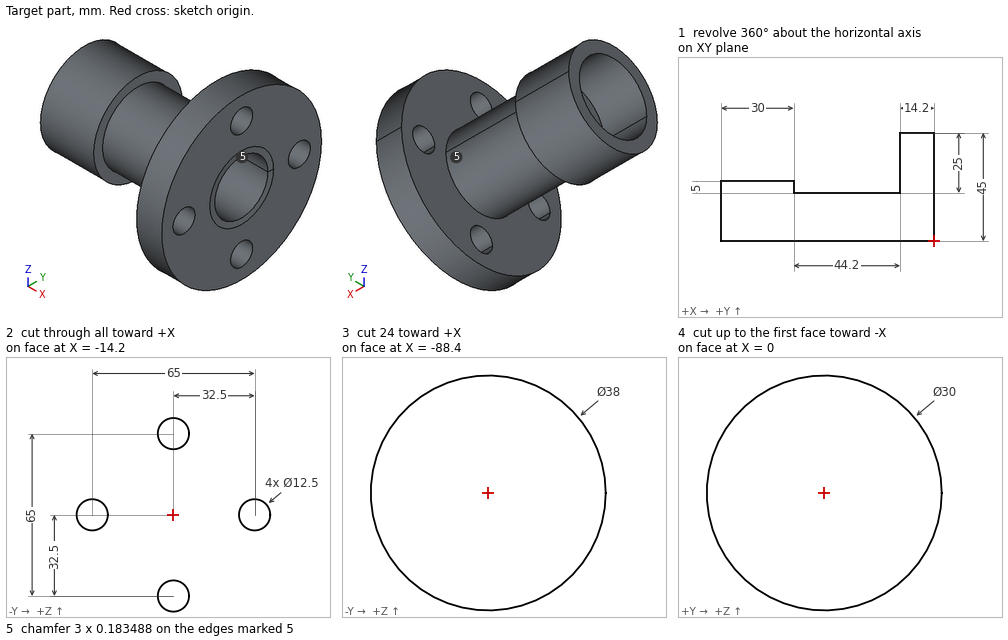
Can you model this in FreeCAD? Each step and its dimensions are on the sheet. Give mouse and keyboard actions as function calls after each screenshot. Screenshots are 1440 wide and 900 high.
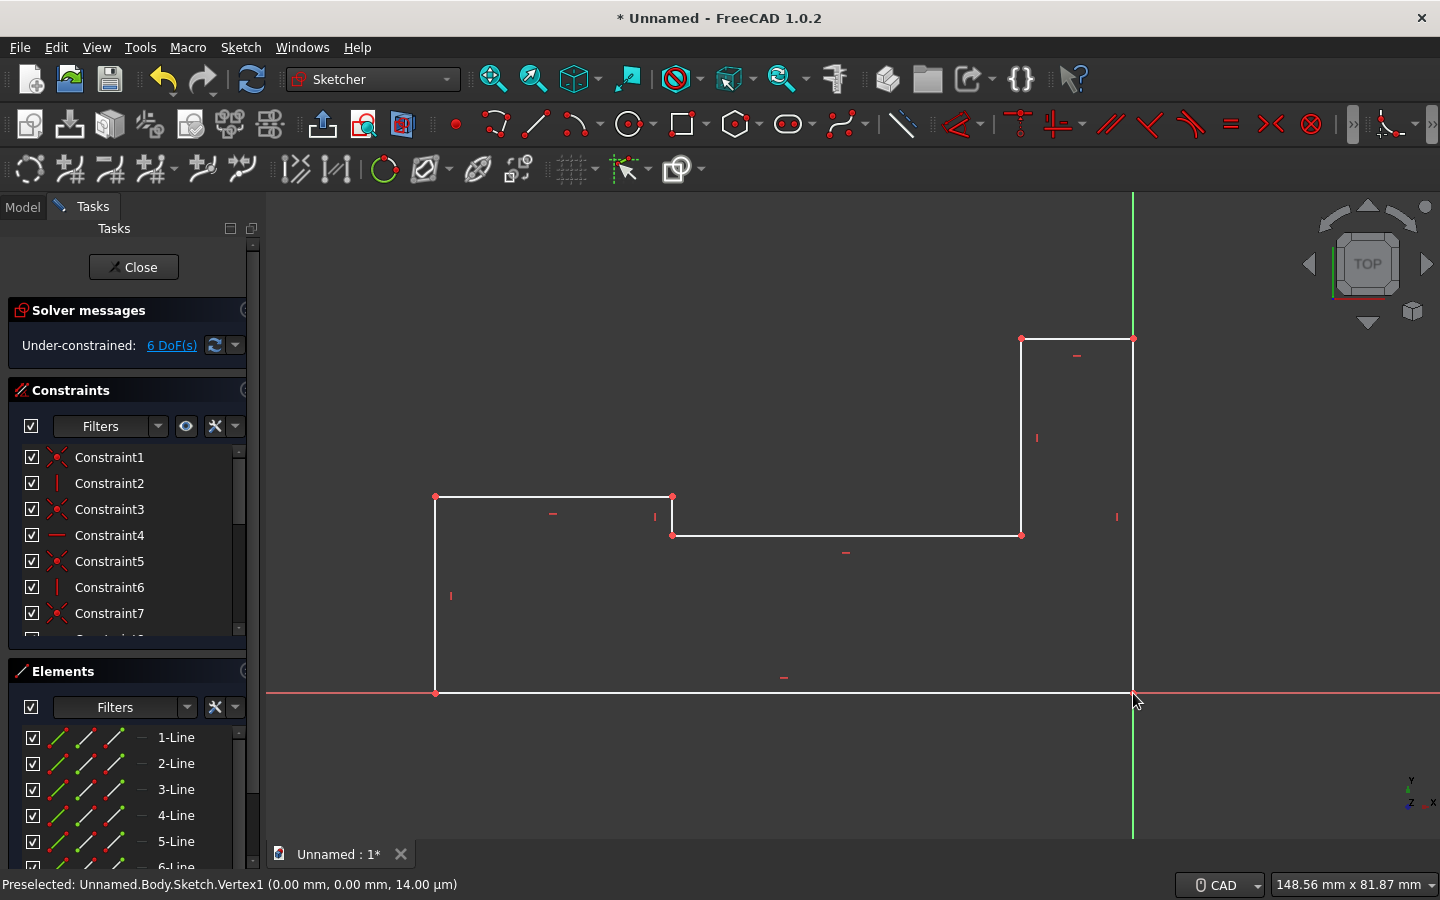
click(956, 124)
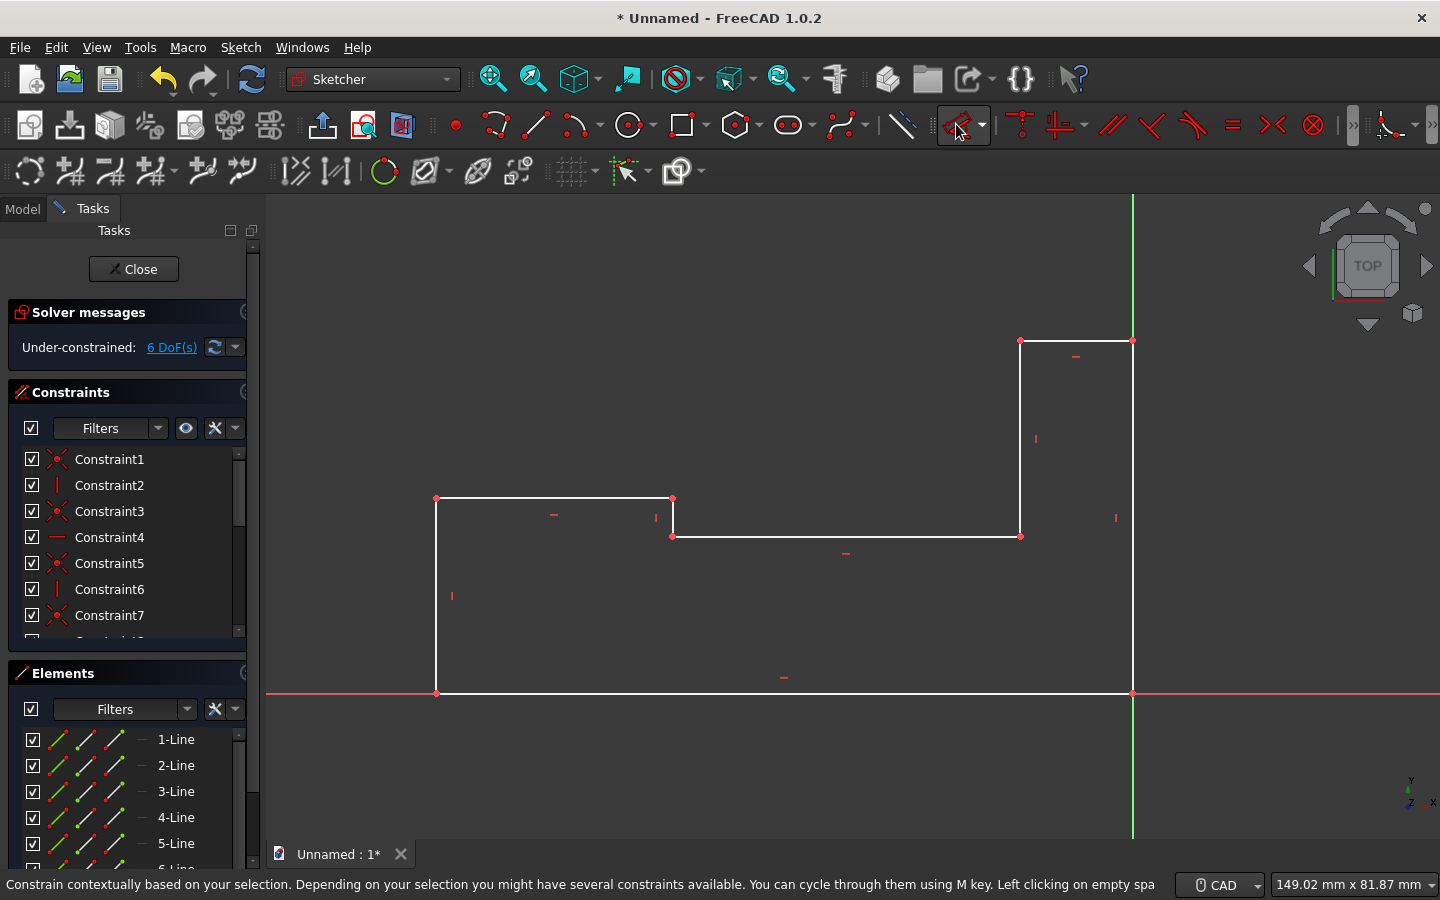
click(673, 525)
click(639, 517)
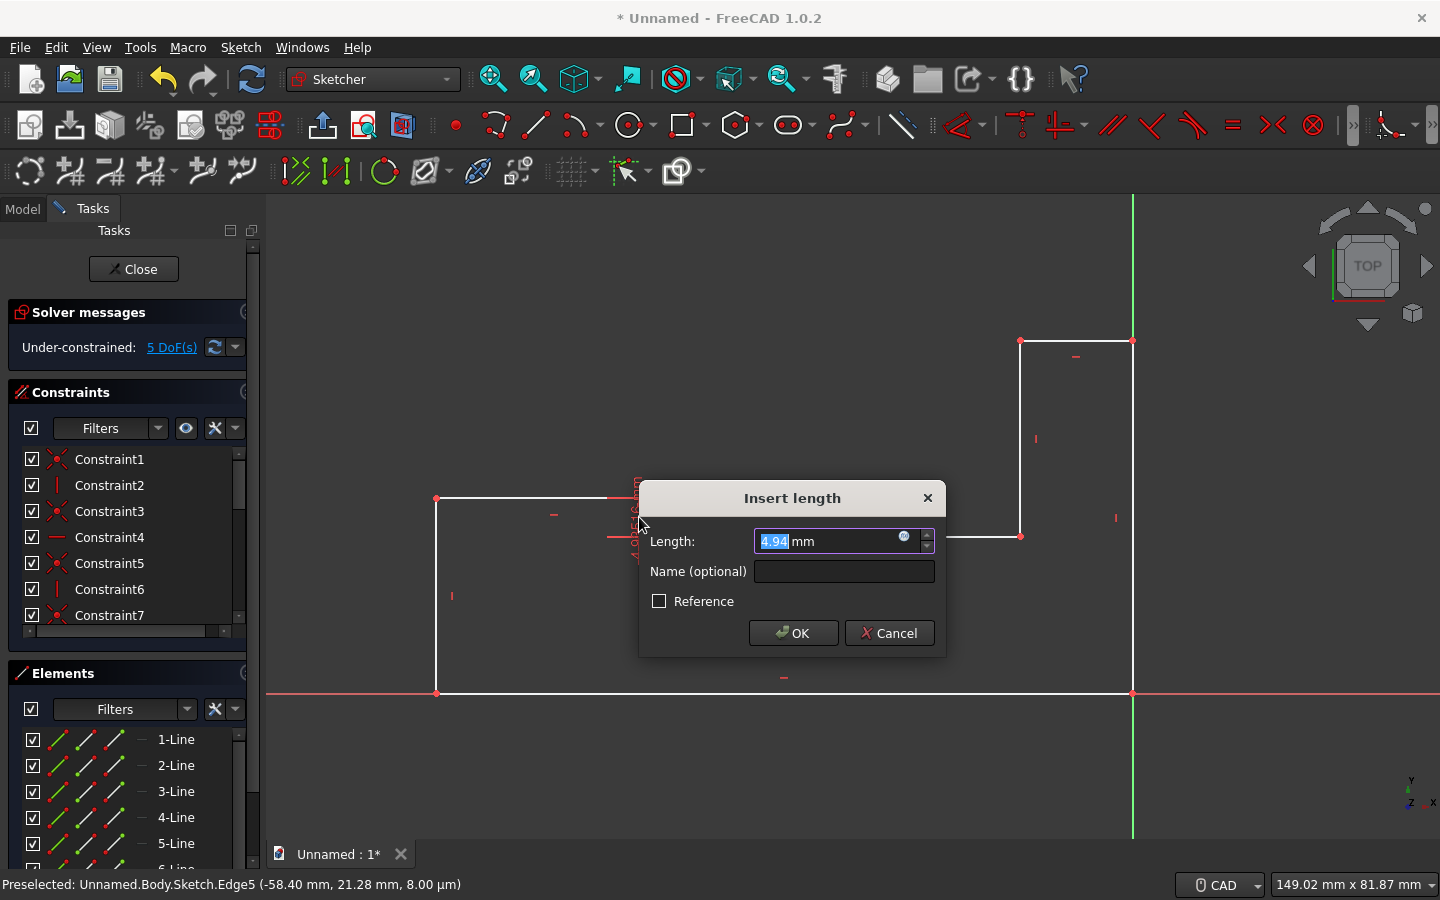
text(5)
key(Return)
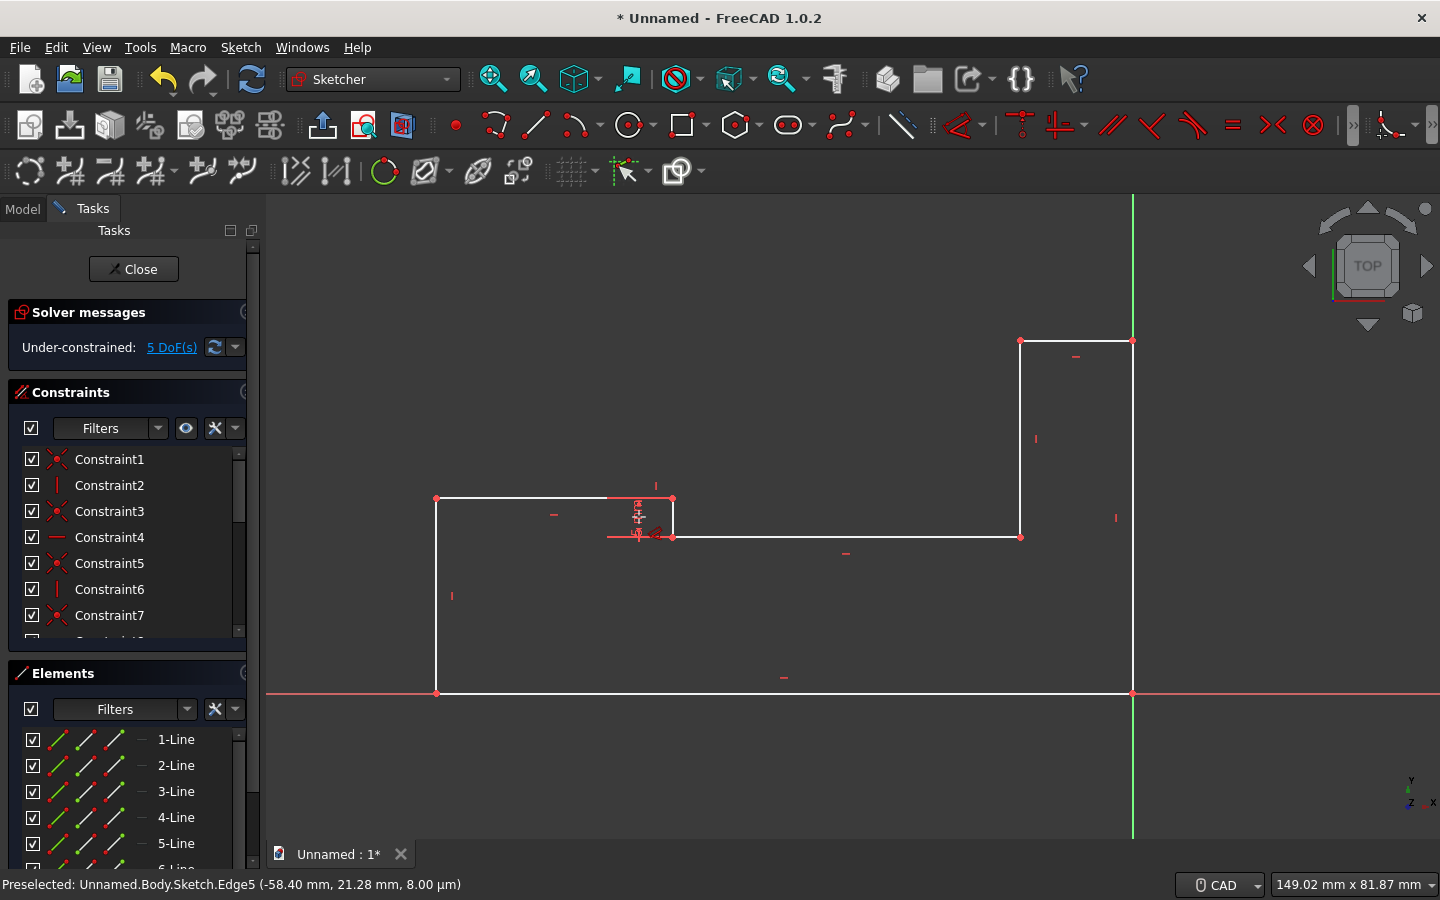
click(1133, 588)
click(1167, 517)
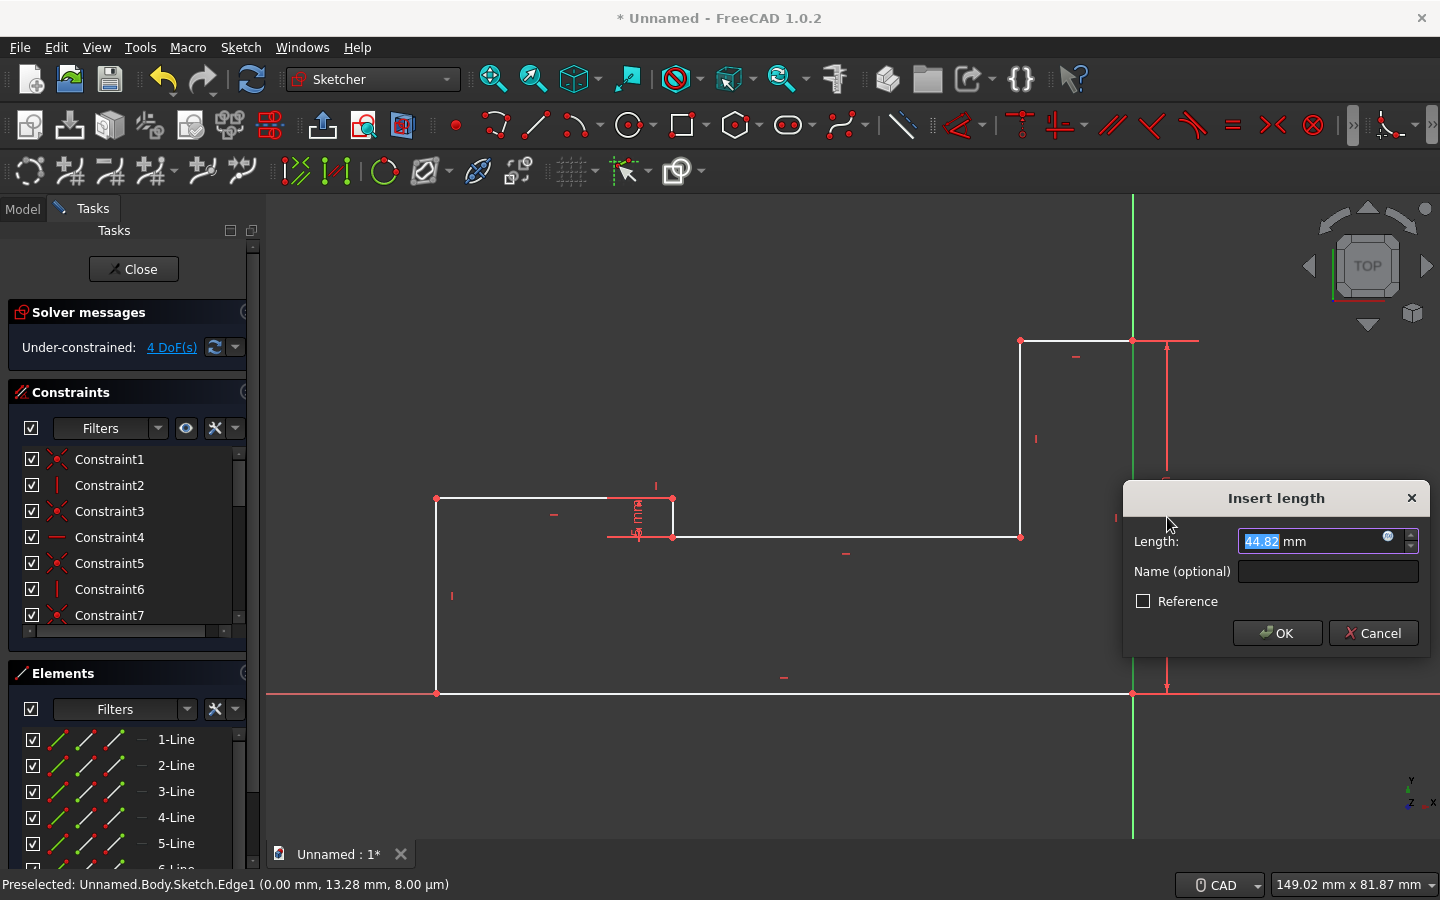
text(45)
key(Return)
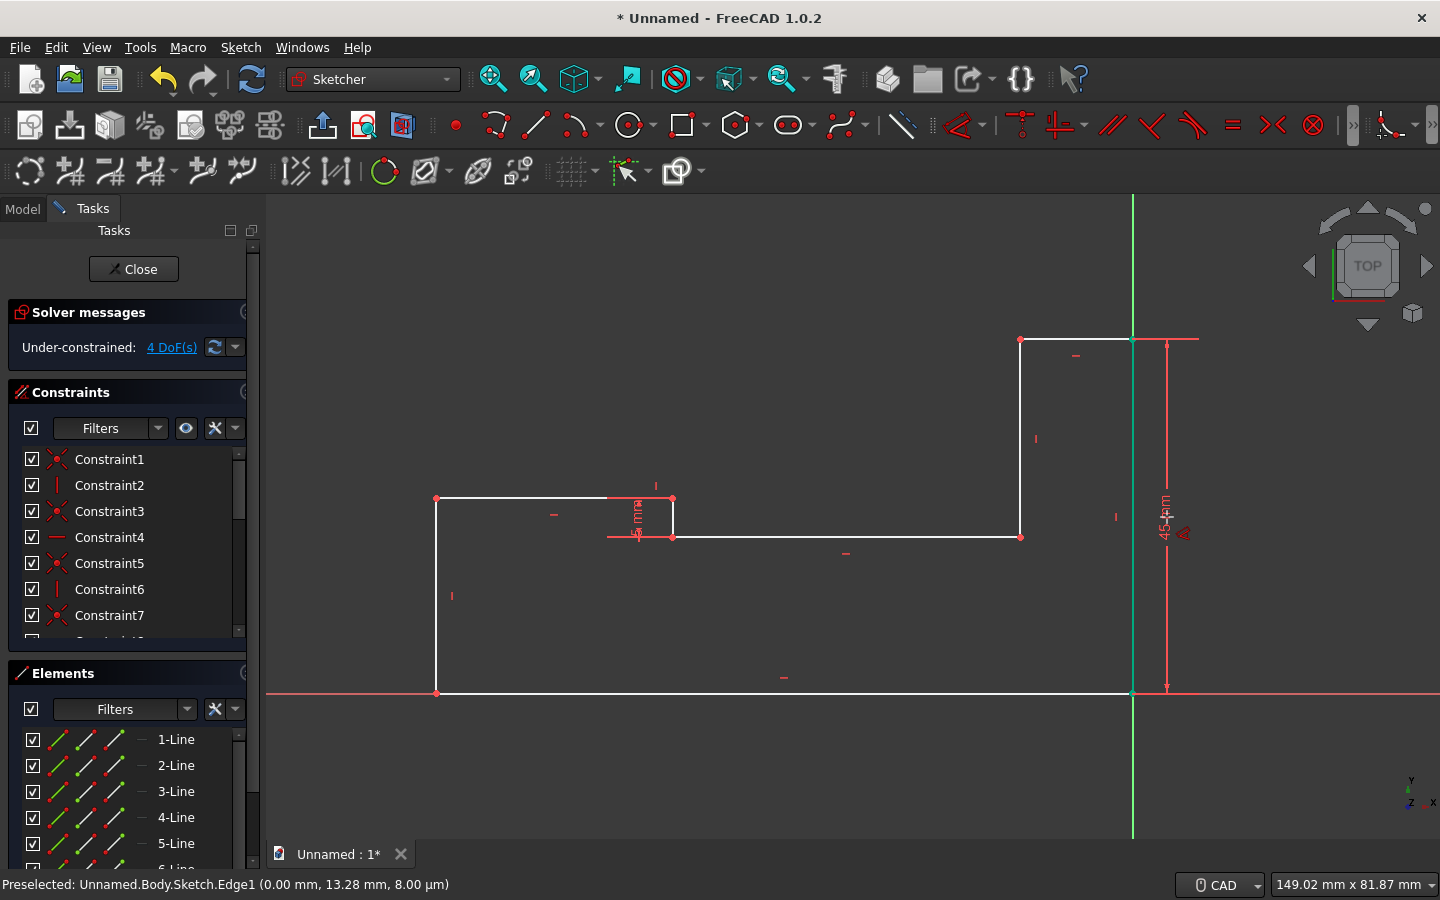
click(1020, 399)
click(1054, 438)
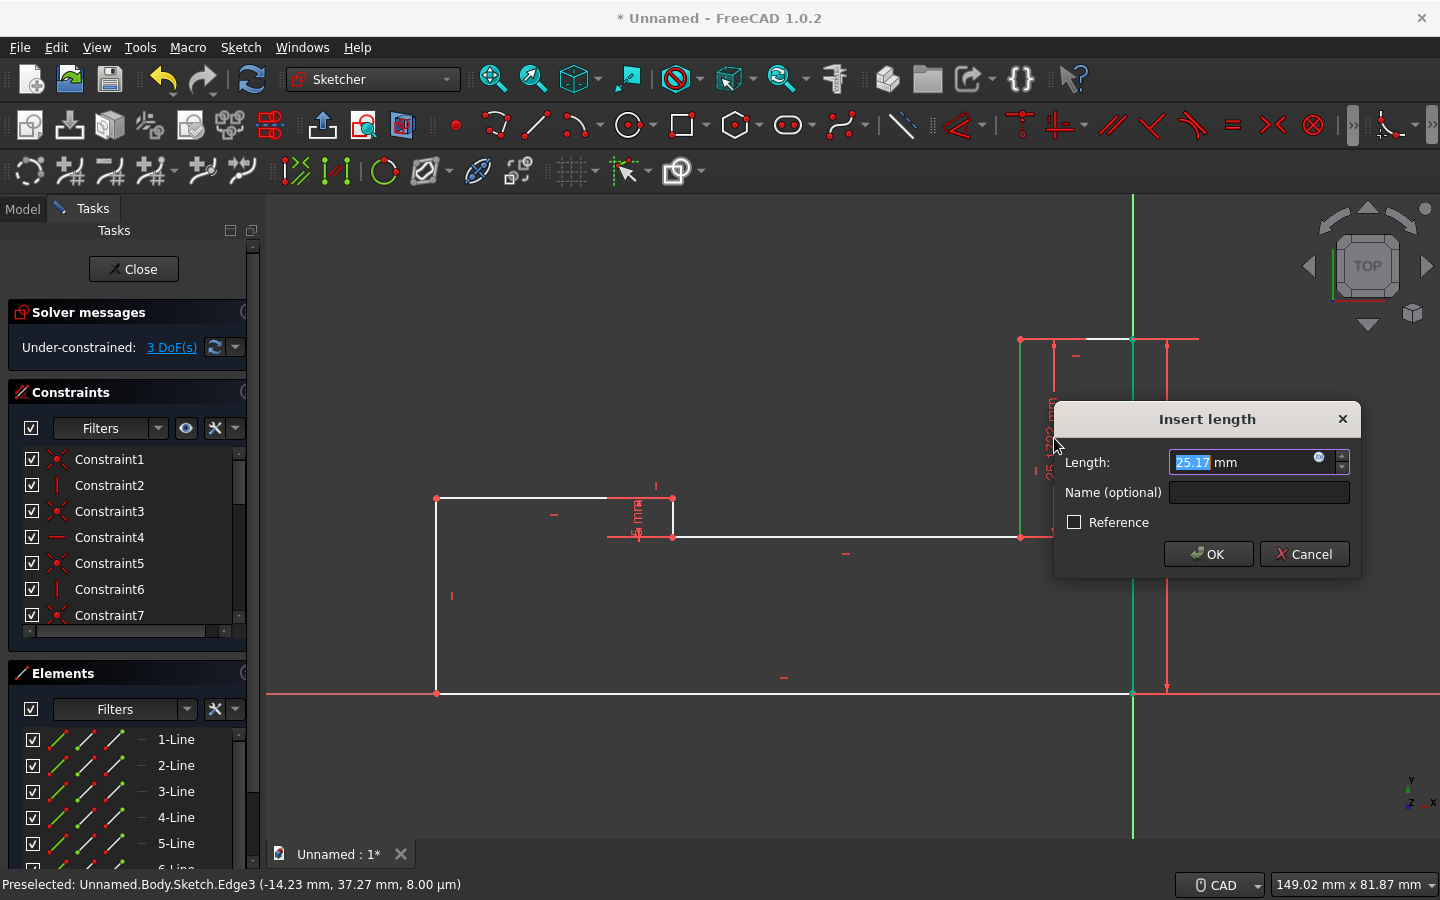
text(25)
key(Return)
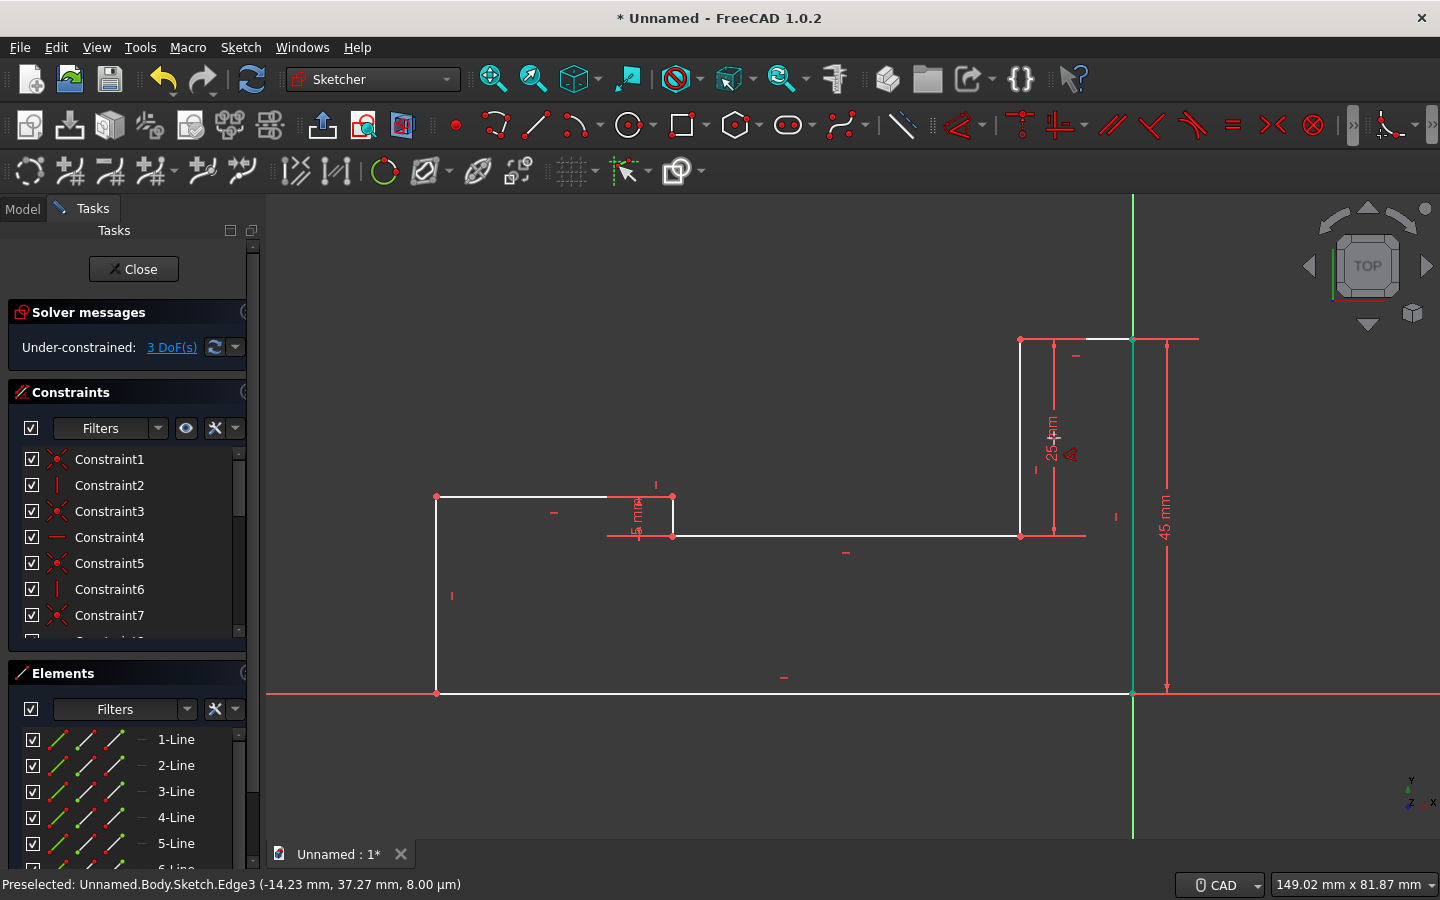
click(602, 497)
click(554, 463)